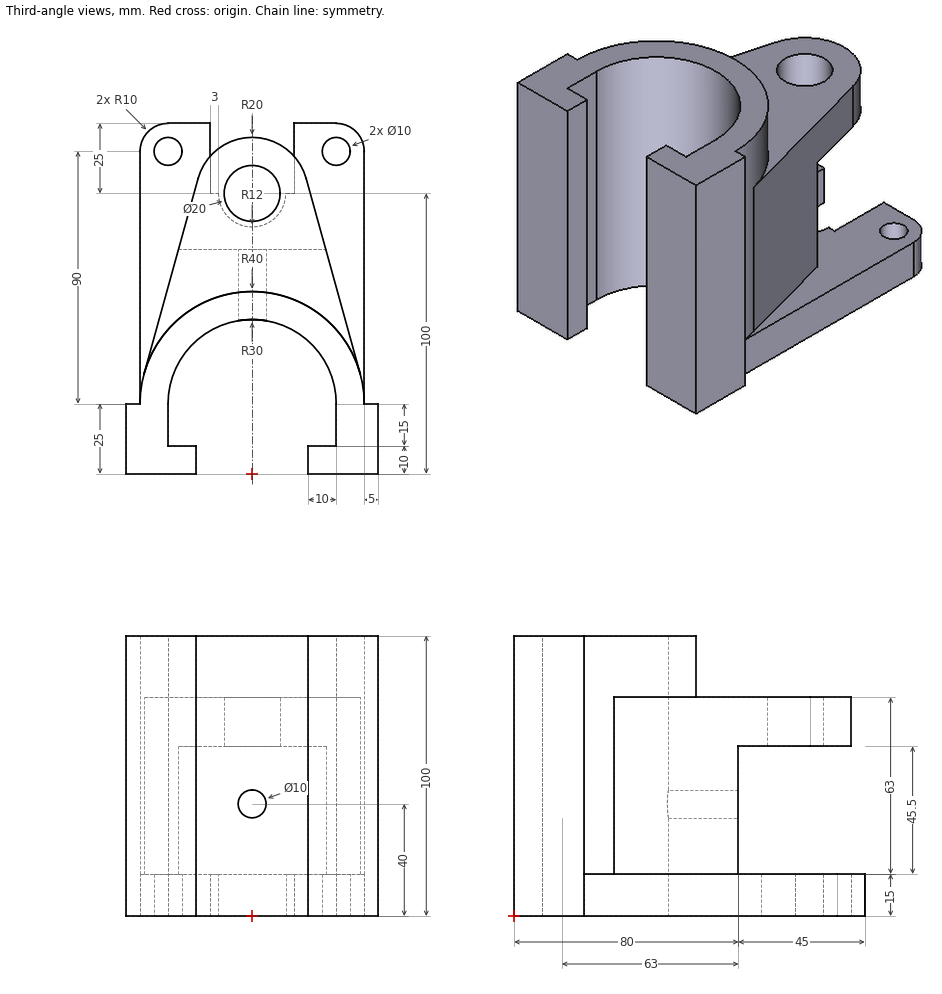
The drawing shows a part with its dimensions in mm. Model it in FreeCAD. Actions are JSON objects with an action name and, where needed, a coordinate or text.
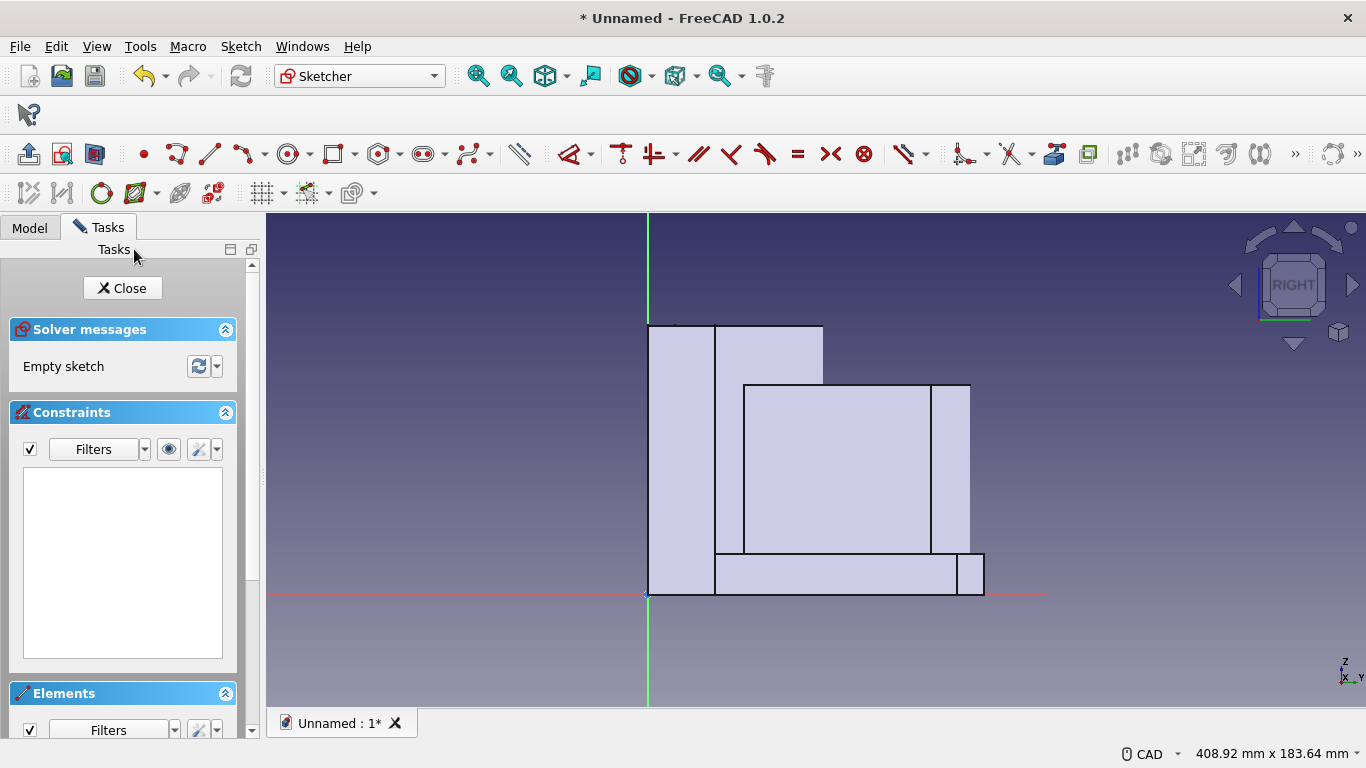
{"action": "key", "text": "q s"}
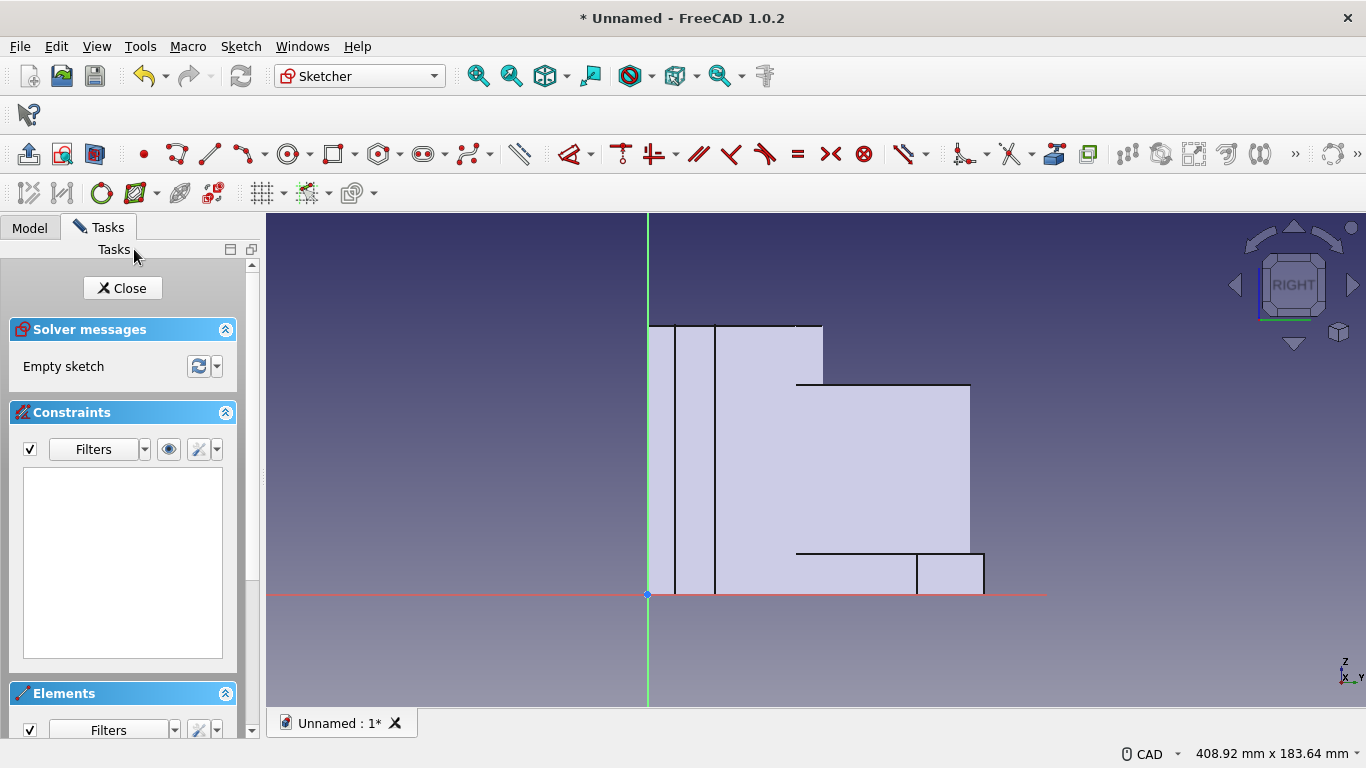
{"action": "scroll", "coordinate": [1026, 512], "scroll_direction": "up", "scroll_amount": 5}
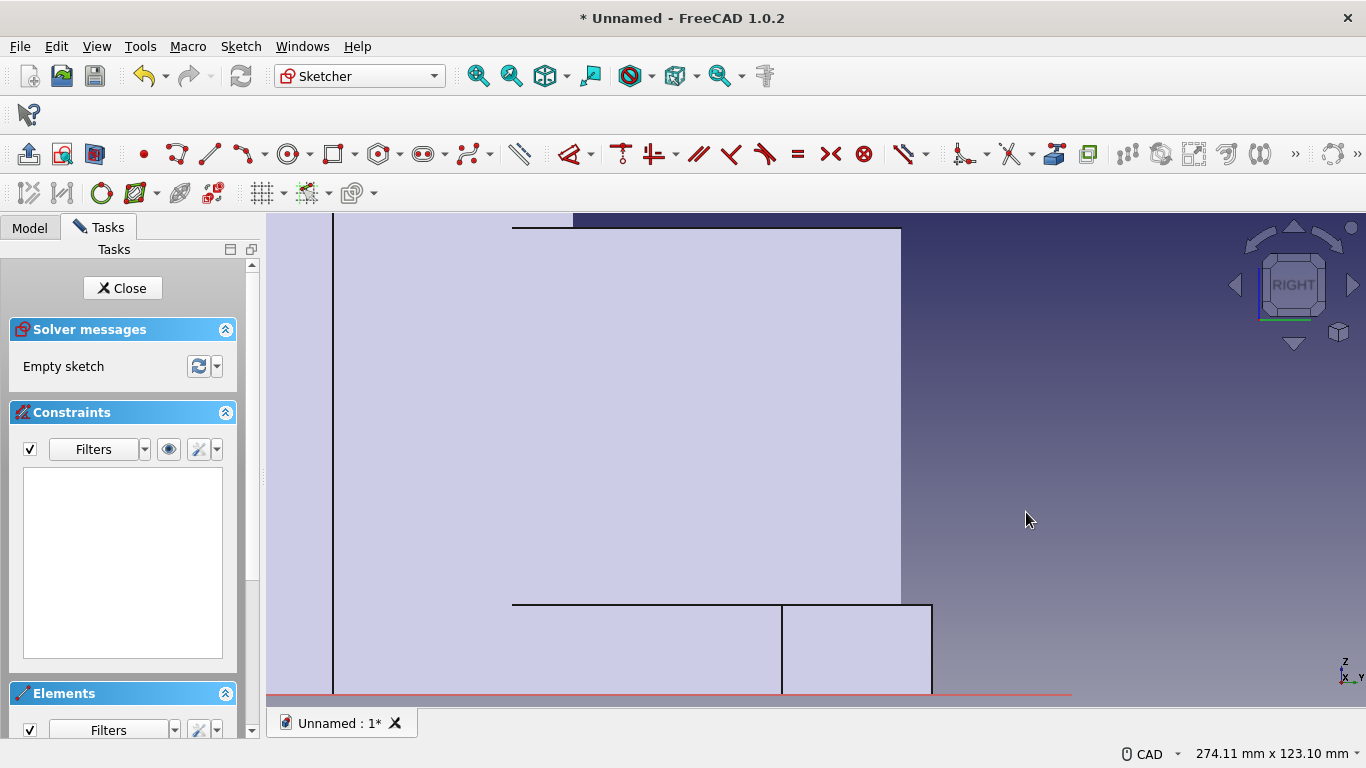
{"action": "key", "text": "g r"}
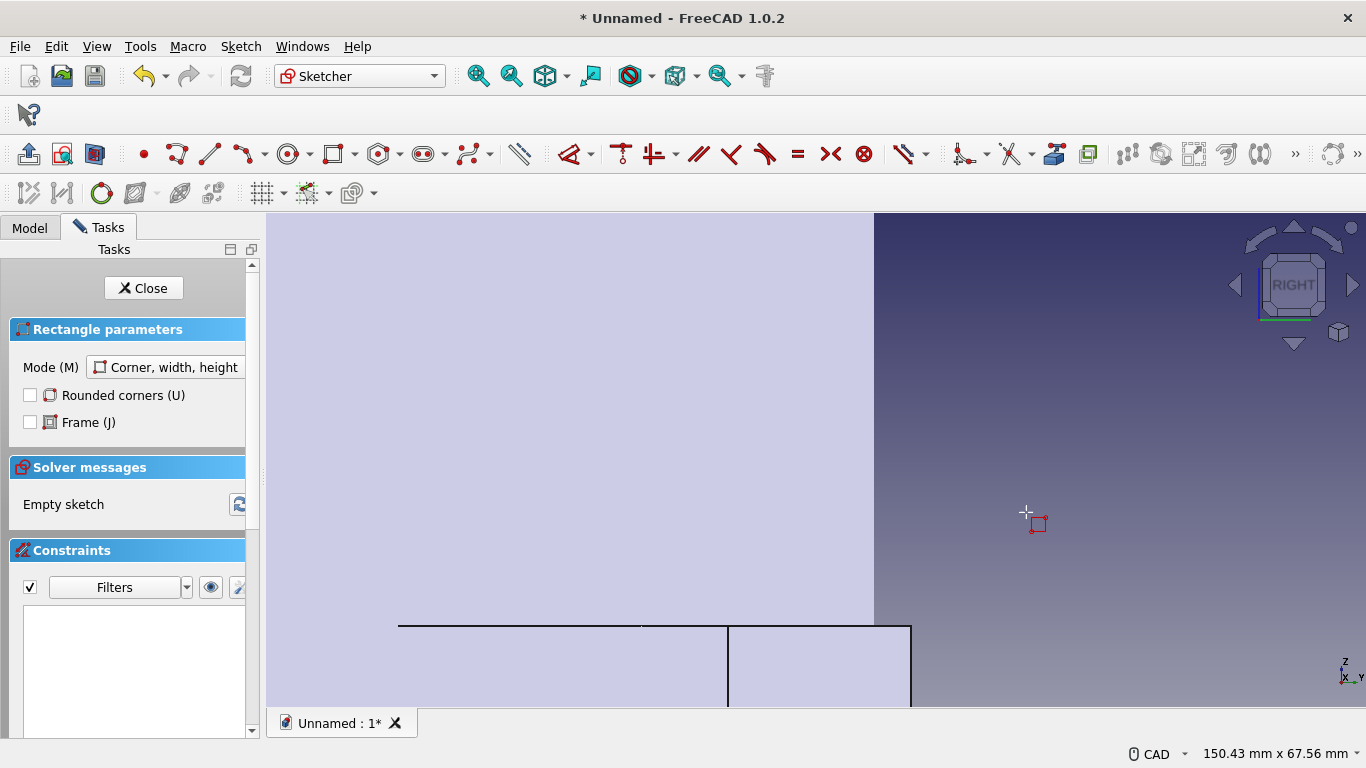
{"action": "left_click", "coordinate": [582, 293]}
{"action": "mouse_move", "coordinate": [911, 626]}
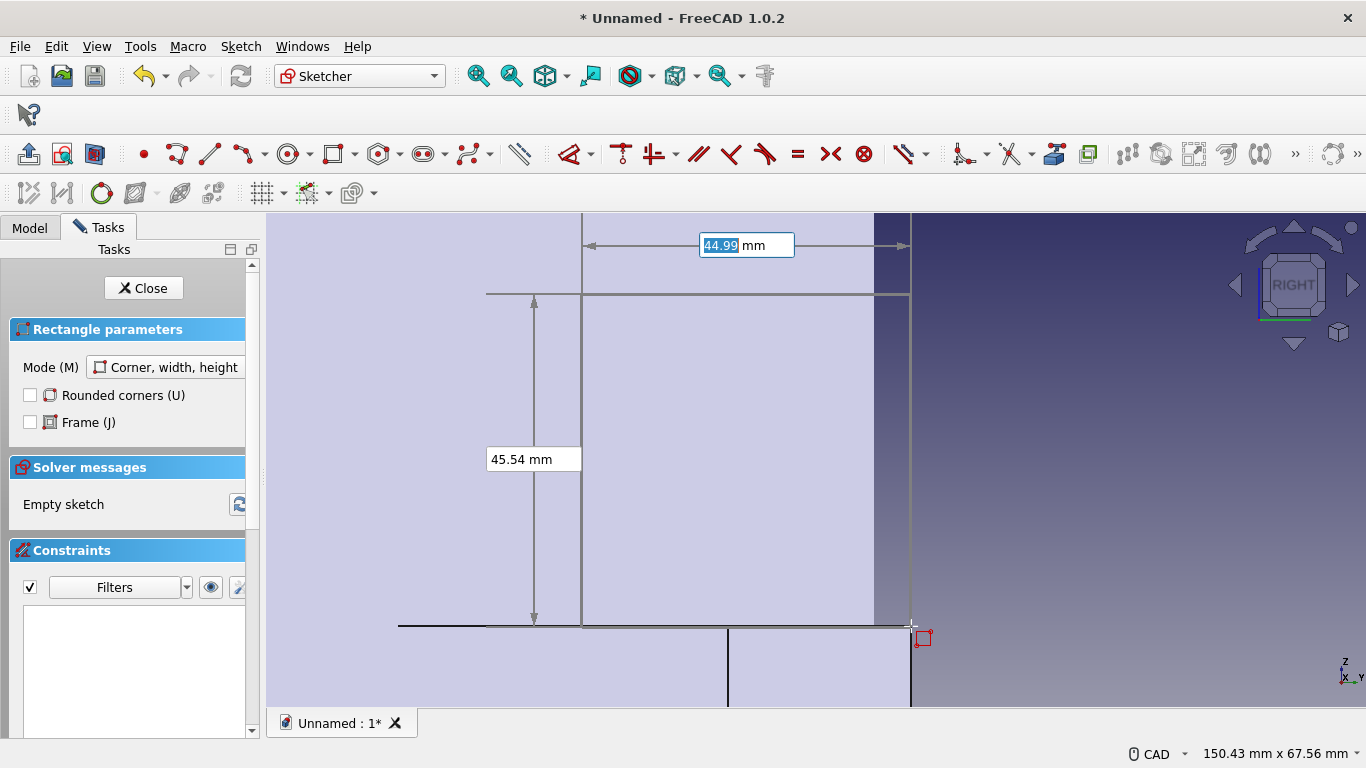
{"action": "type", "text": "45"}
{"action": "key", "text": "Tab"}
{"action": "type", "text": "45.5"}
{"action": "key", "text": "Return"}
{"action": "key", "text": "Escape"}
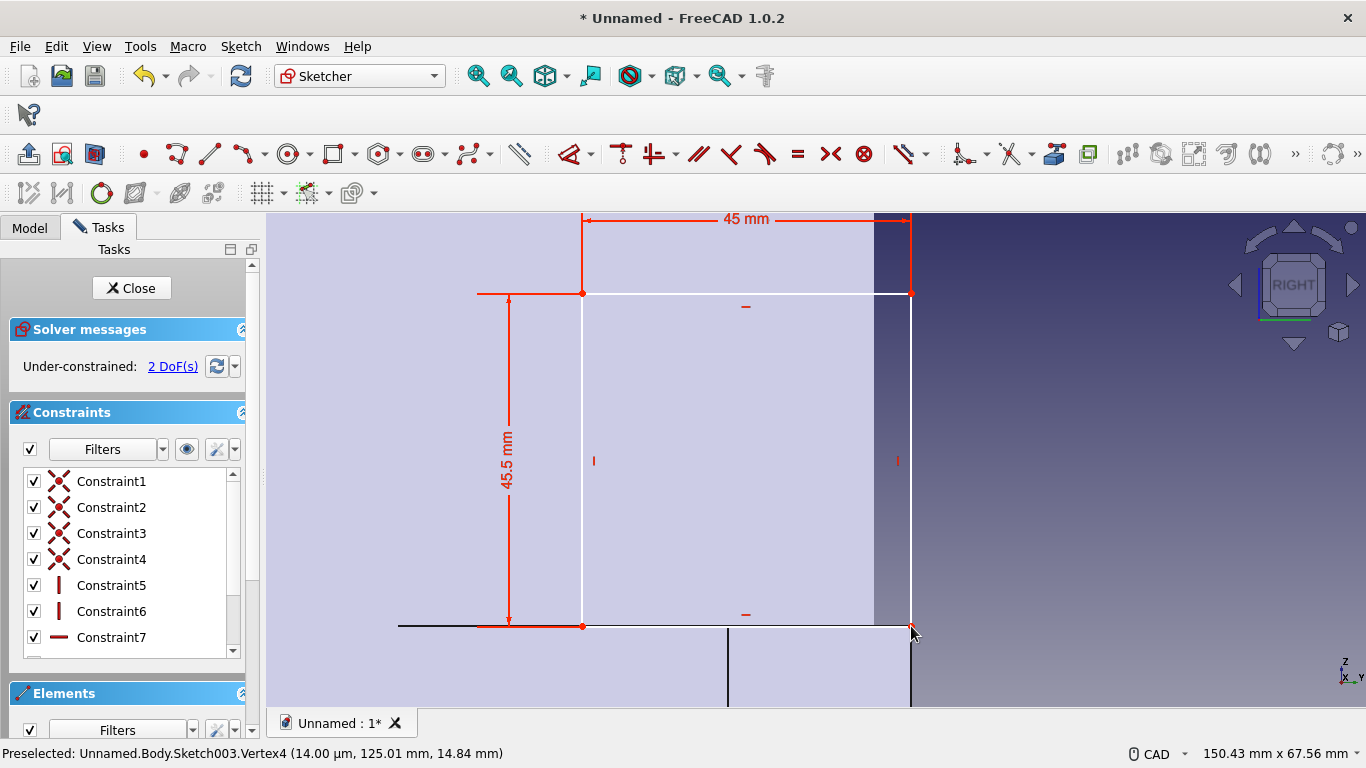
{"action": "key", "text": "d"}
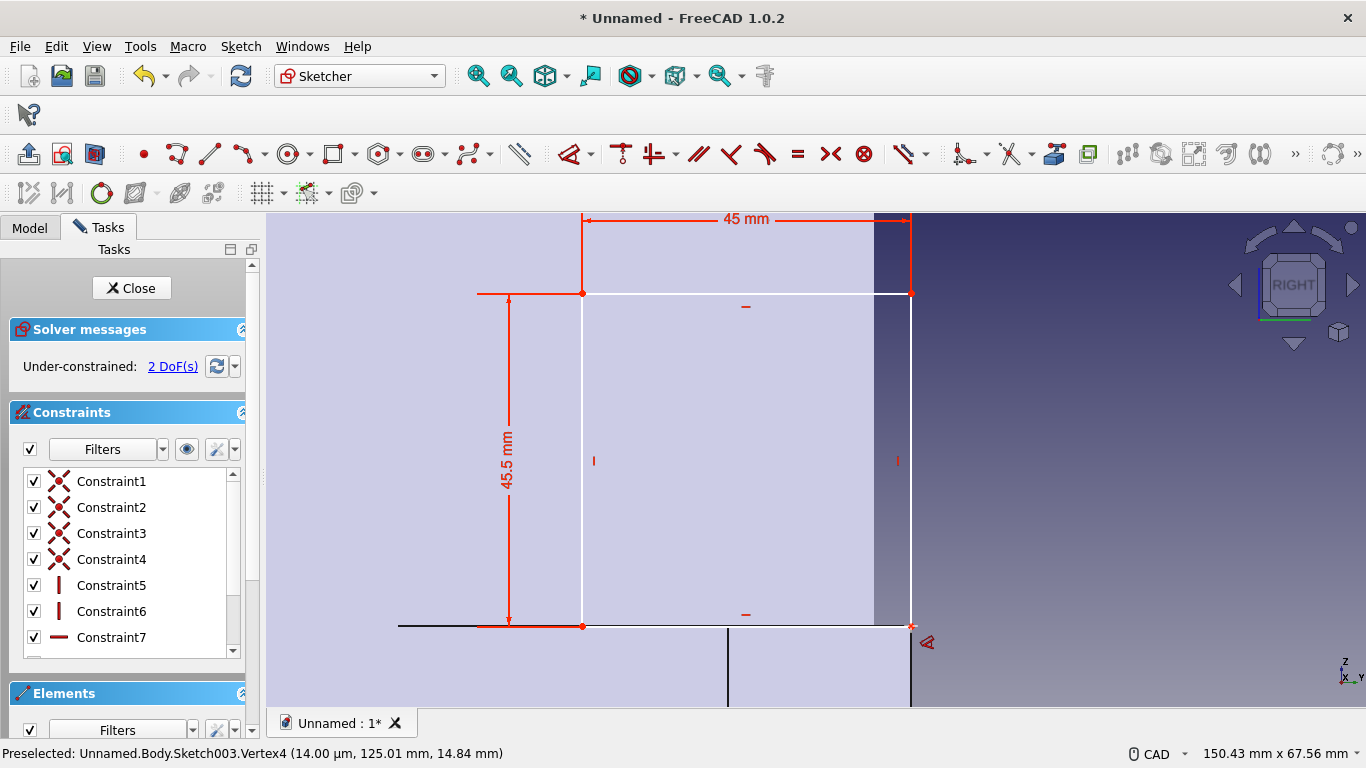
{"action": "left_click", "coordinate": [582, 294]}
{"action": "left_click", "coordinate": [438, 260]}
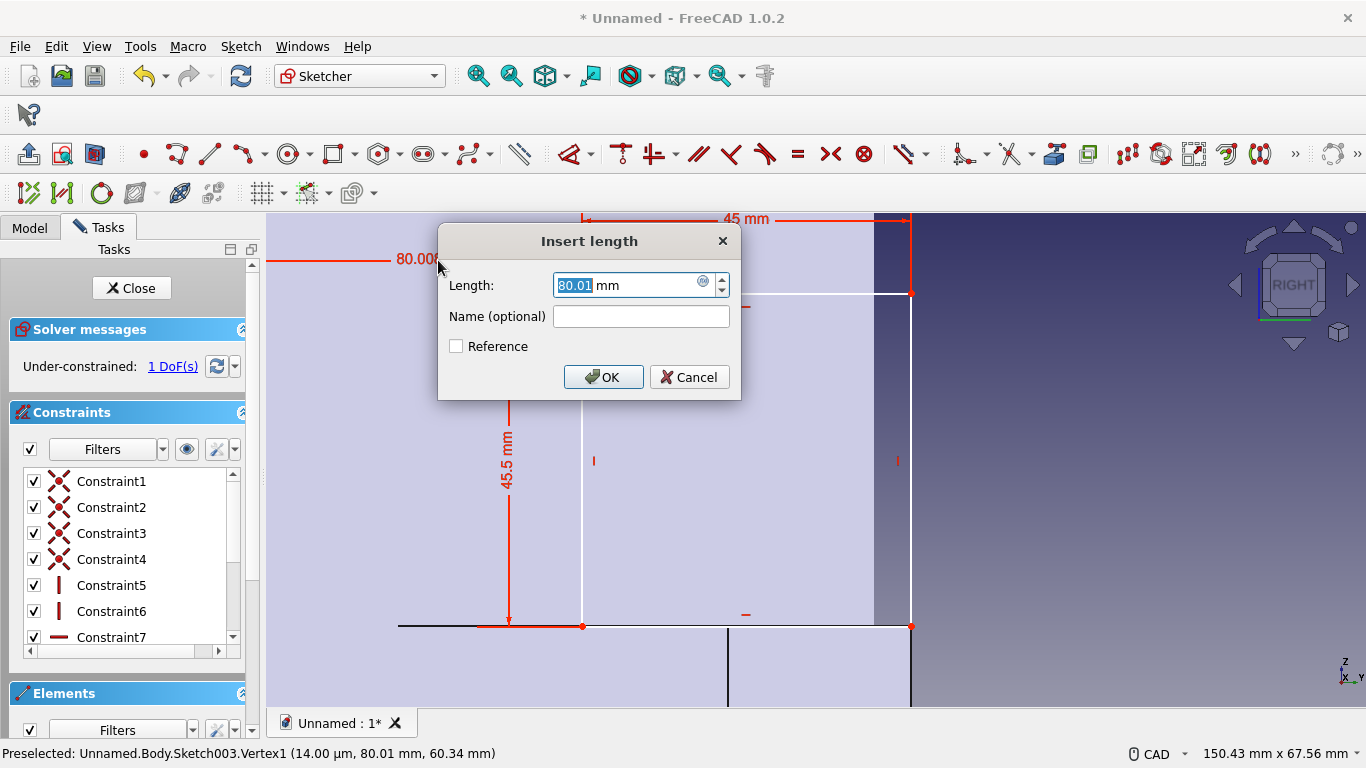
{"action": "type", "text": "80"}
{"action": "key", "text": "Return"}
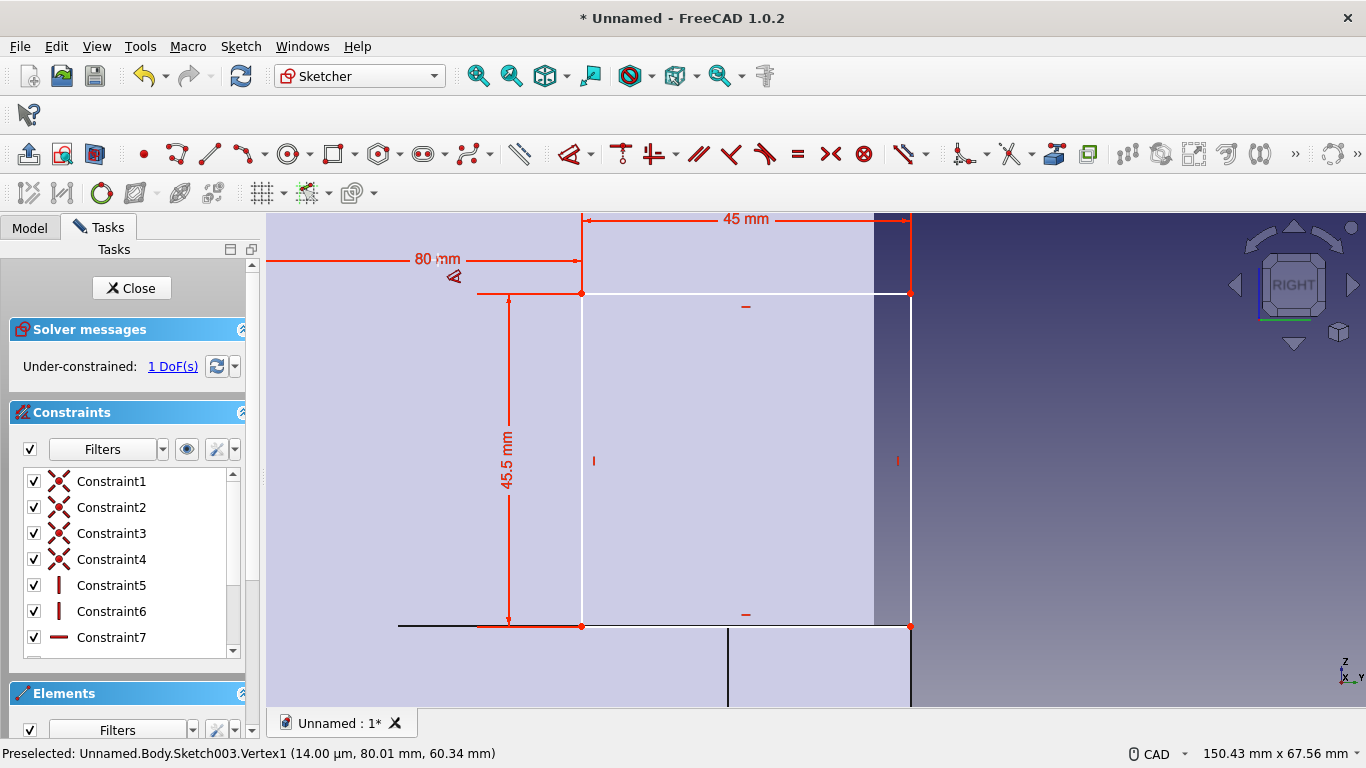
{"action": "left_click", "coordinate": [582, 627]}
{"action": "left_click", "coordinate": [616, 653]}